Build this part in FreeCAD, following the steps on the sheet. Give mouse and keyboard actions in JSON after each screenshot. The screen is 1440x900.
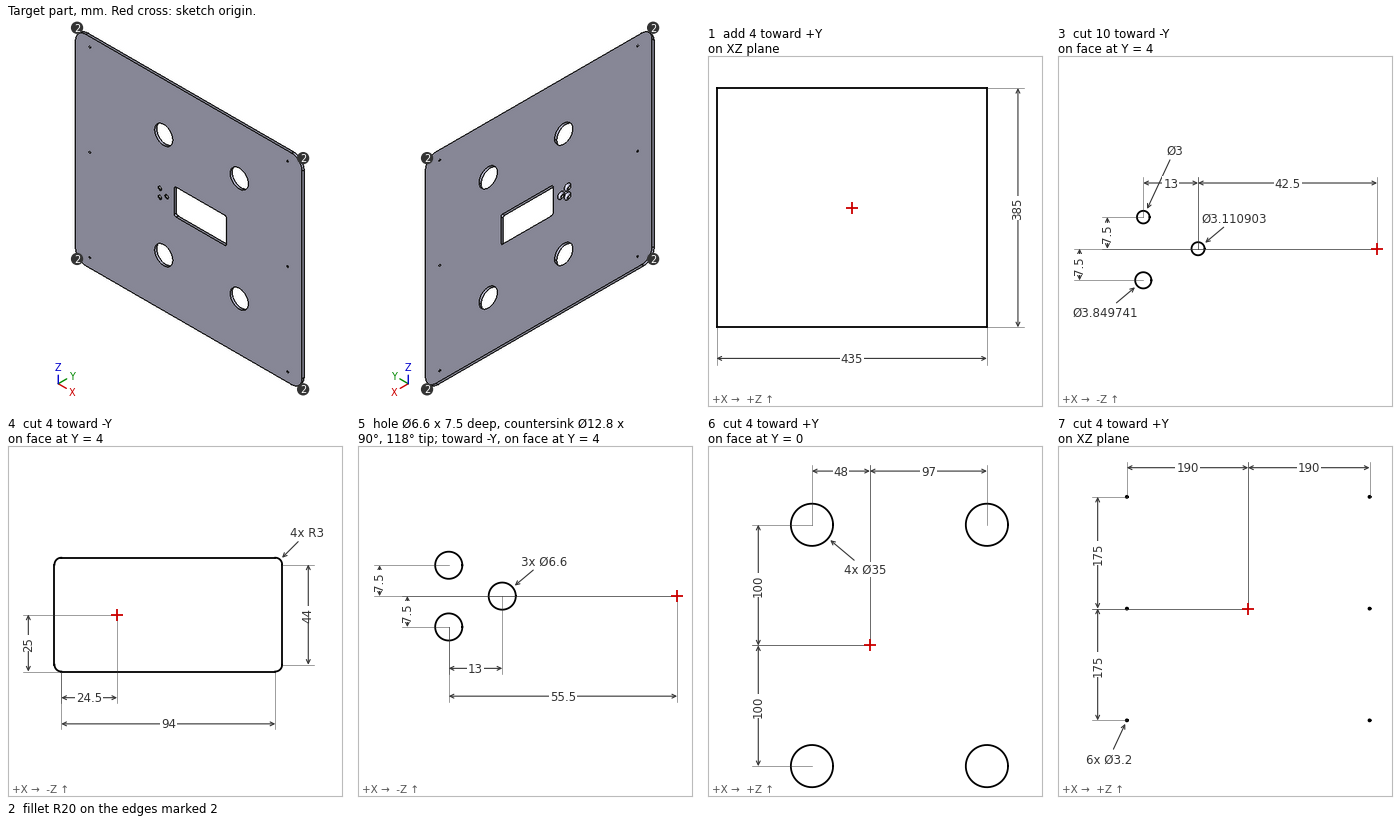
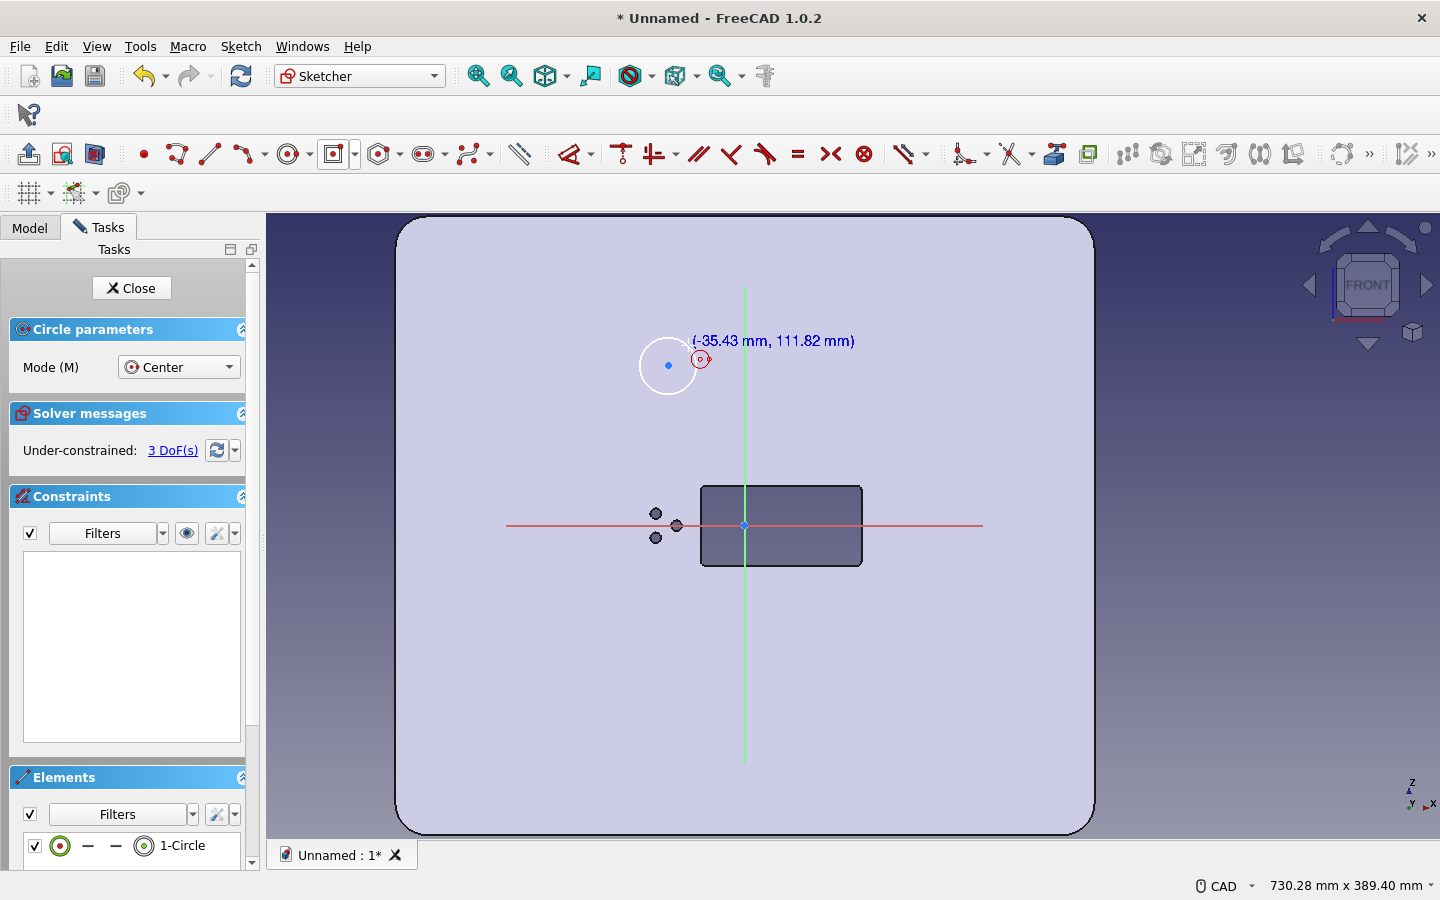
{"action": "left_click", "coordinate": [901, 365]}
{"action": "left_click", "coordinate": [921, 345]}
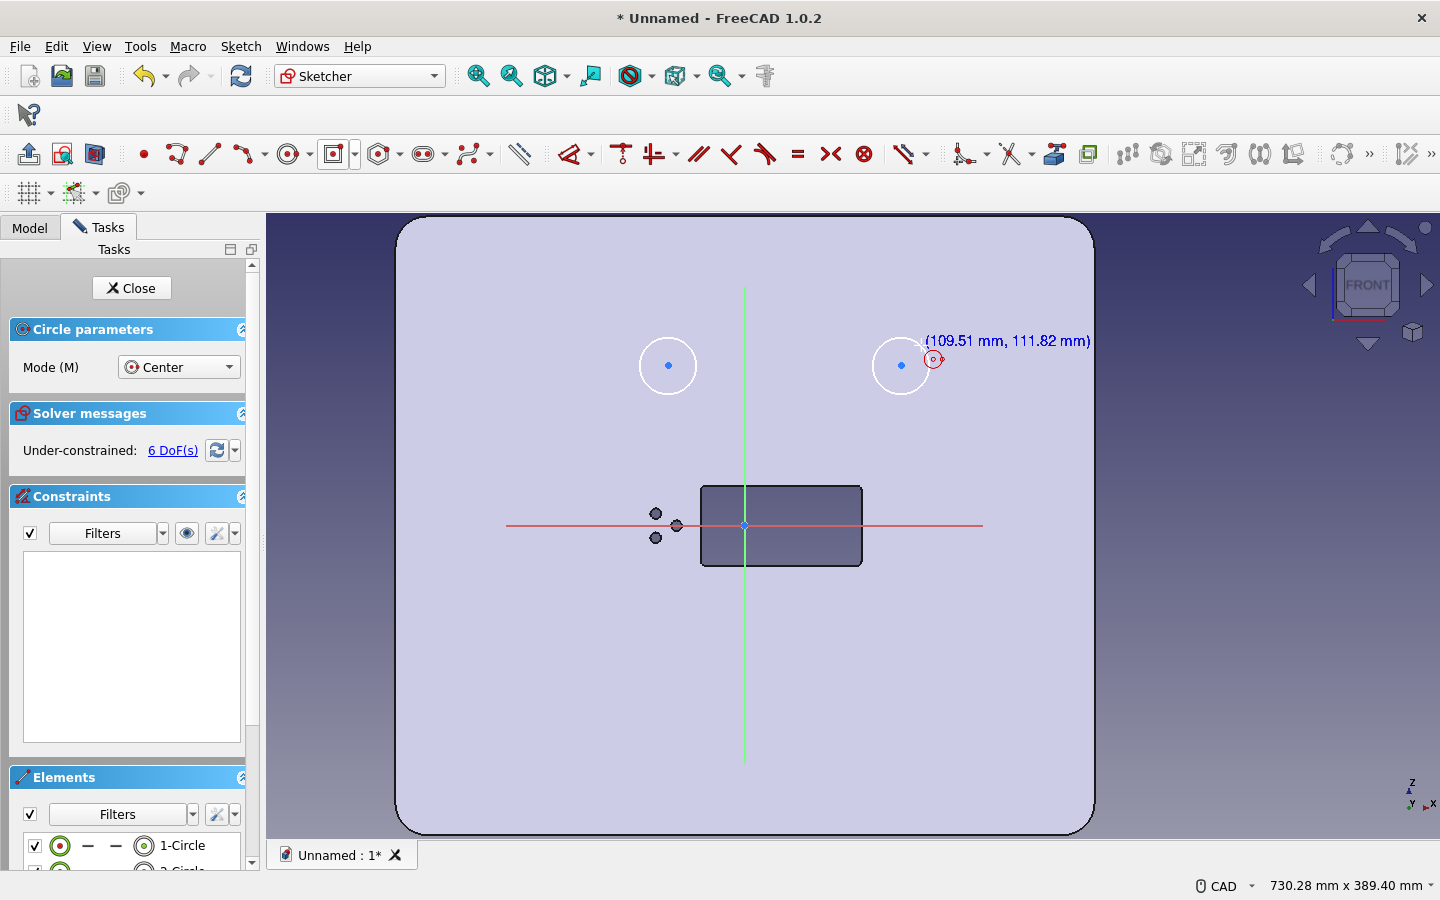
{"action": "left_click", "coordinate": [668, 687]}
{"action": "left_click", "coordinate": [688, 667]}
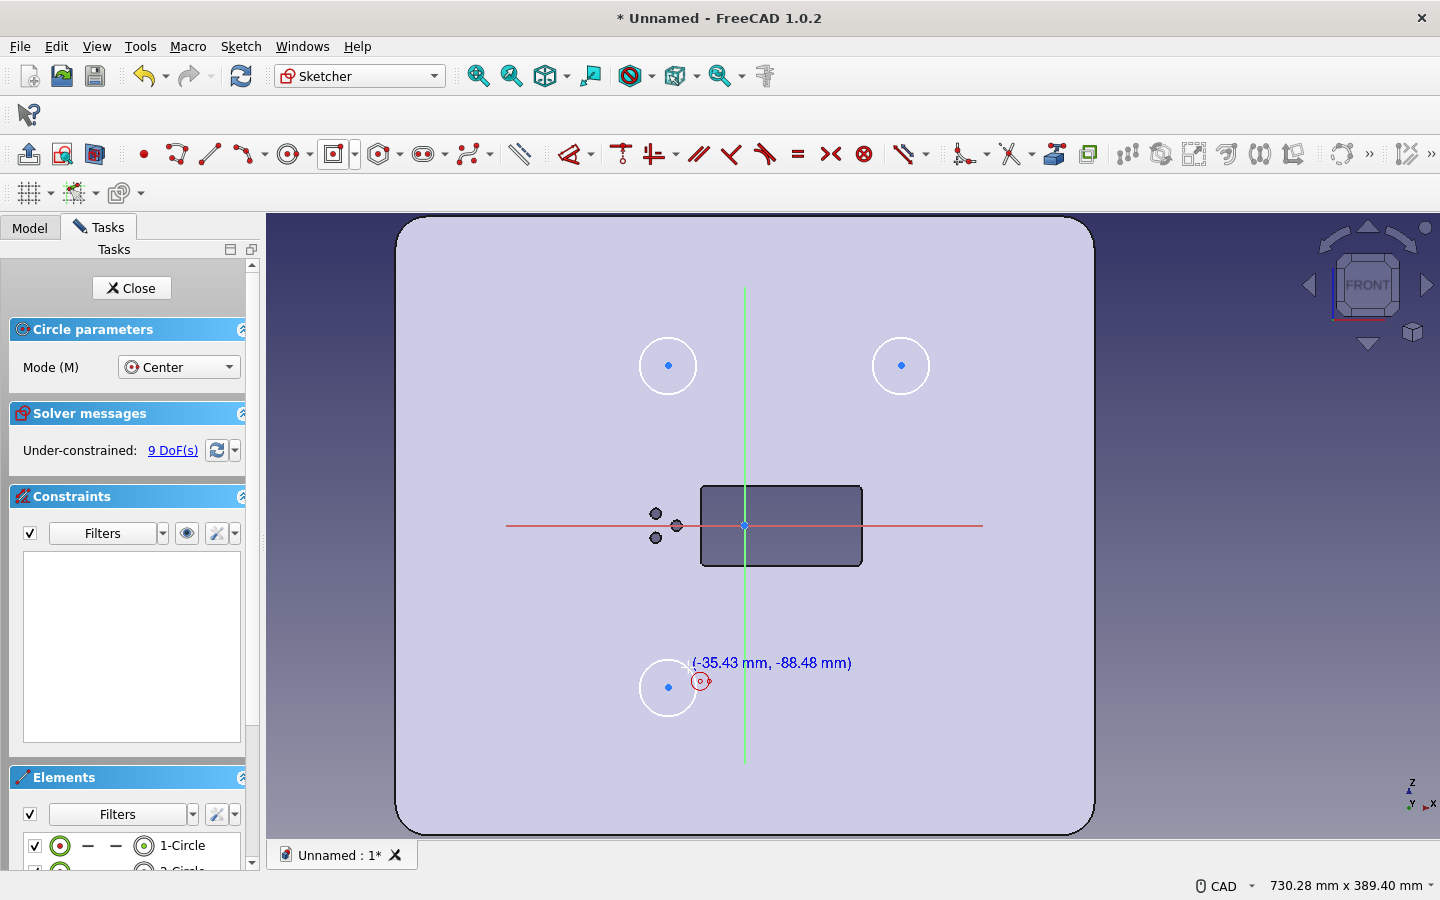
{"action": "left_click", "coordinate": [901, 687]}
{"action": "left_click", "coordinate": [921, 667]}
{"action": "key", "text": "Escape"}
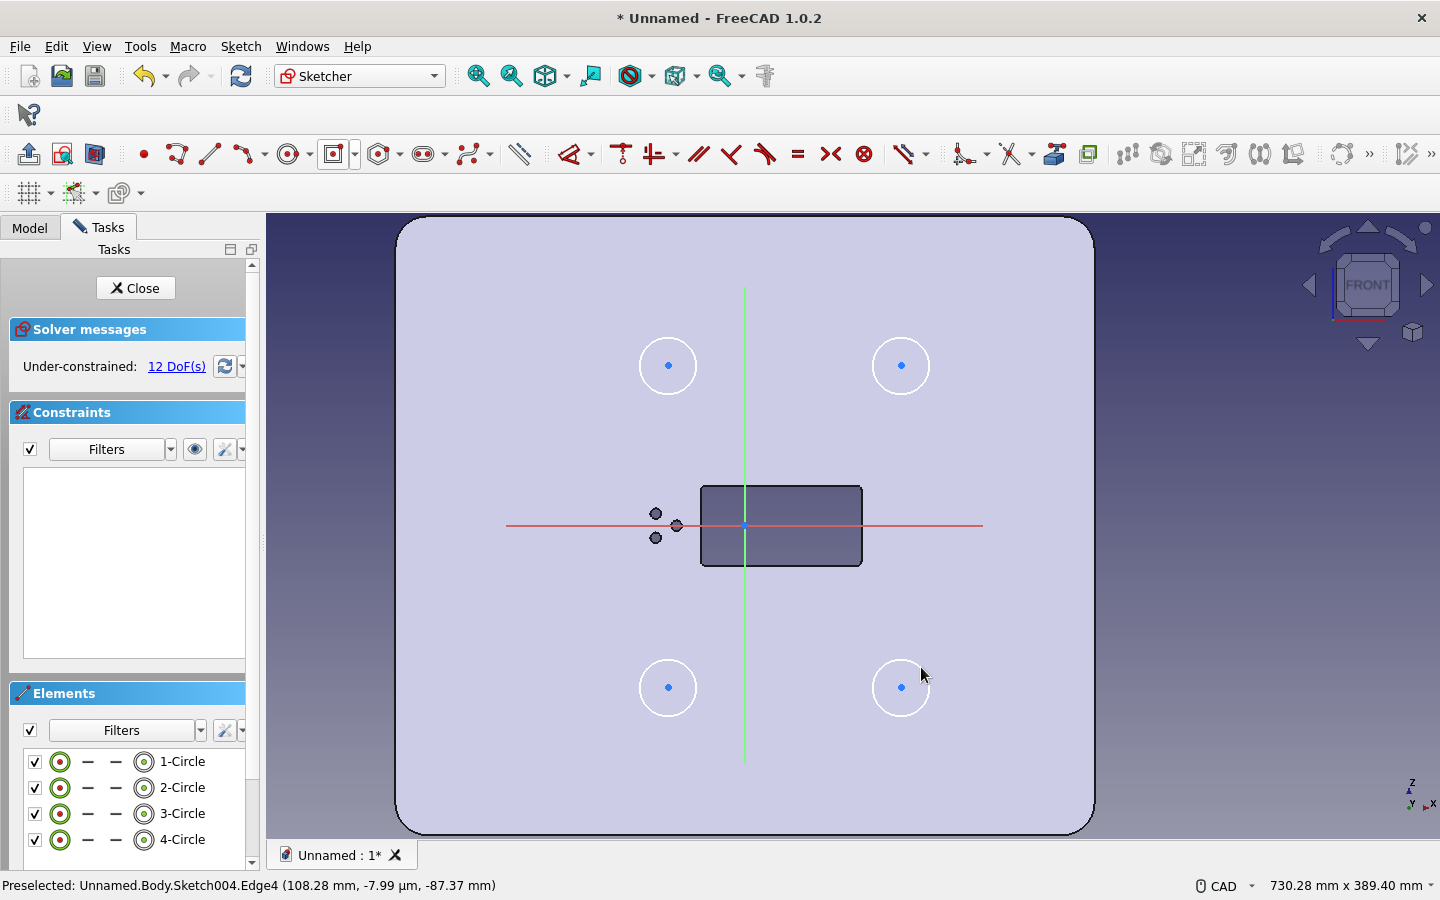
{"action": "left_click", "coordinate": [688, 346]}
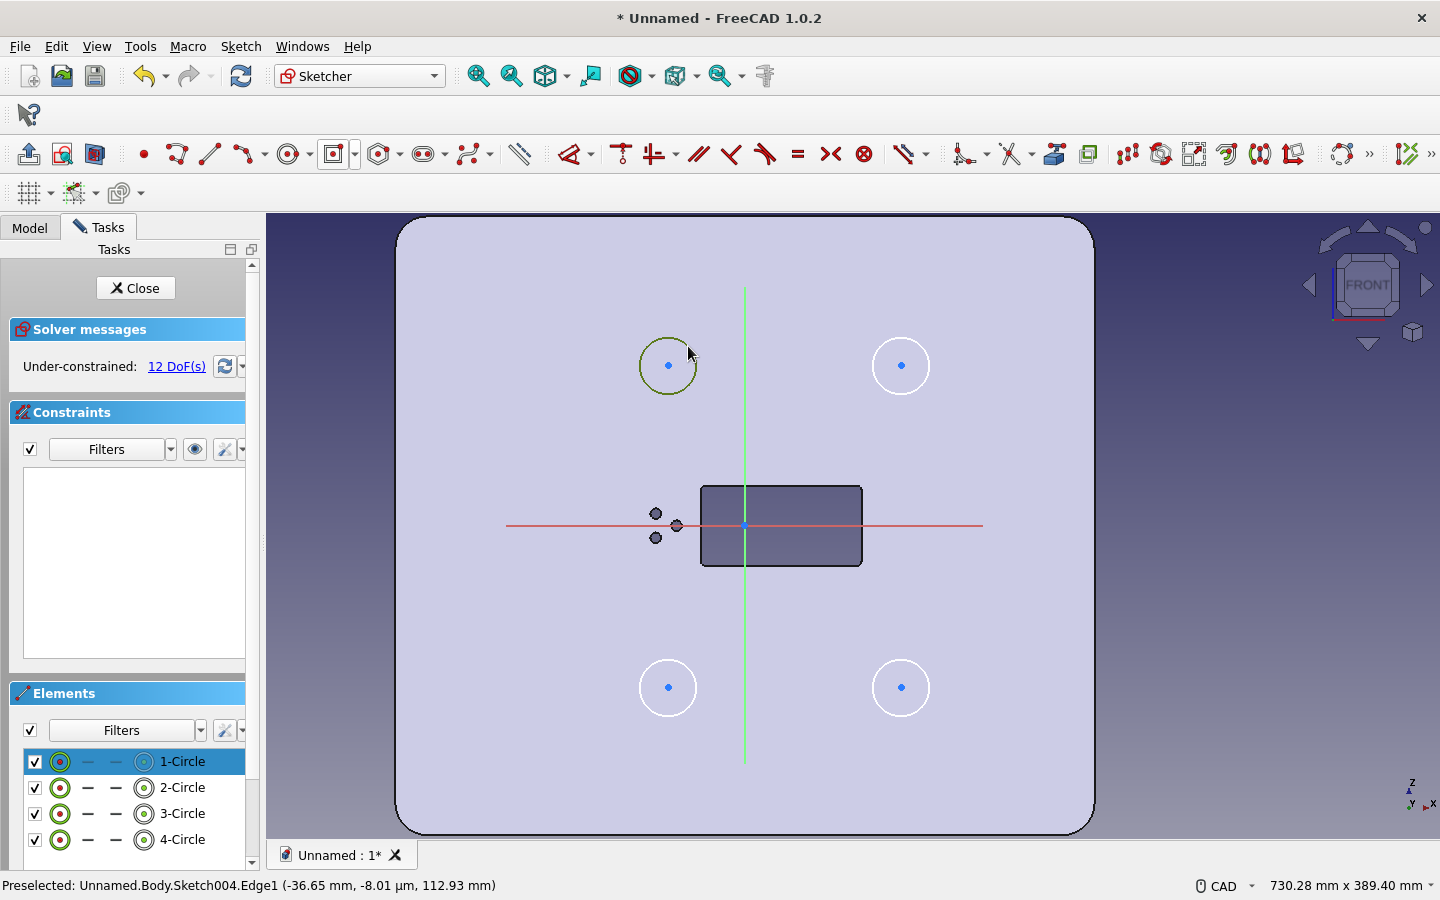
{"action": "left_click", "coordinate": [921, 346]}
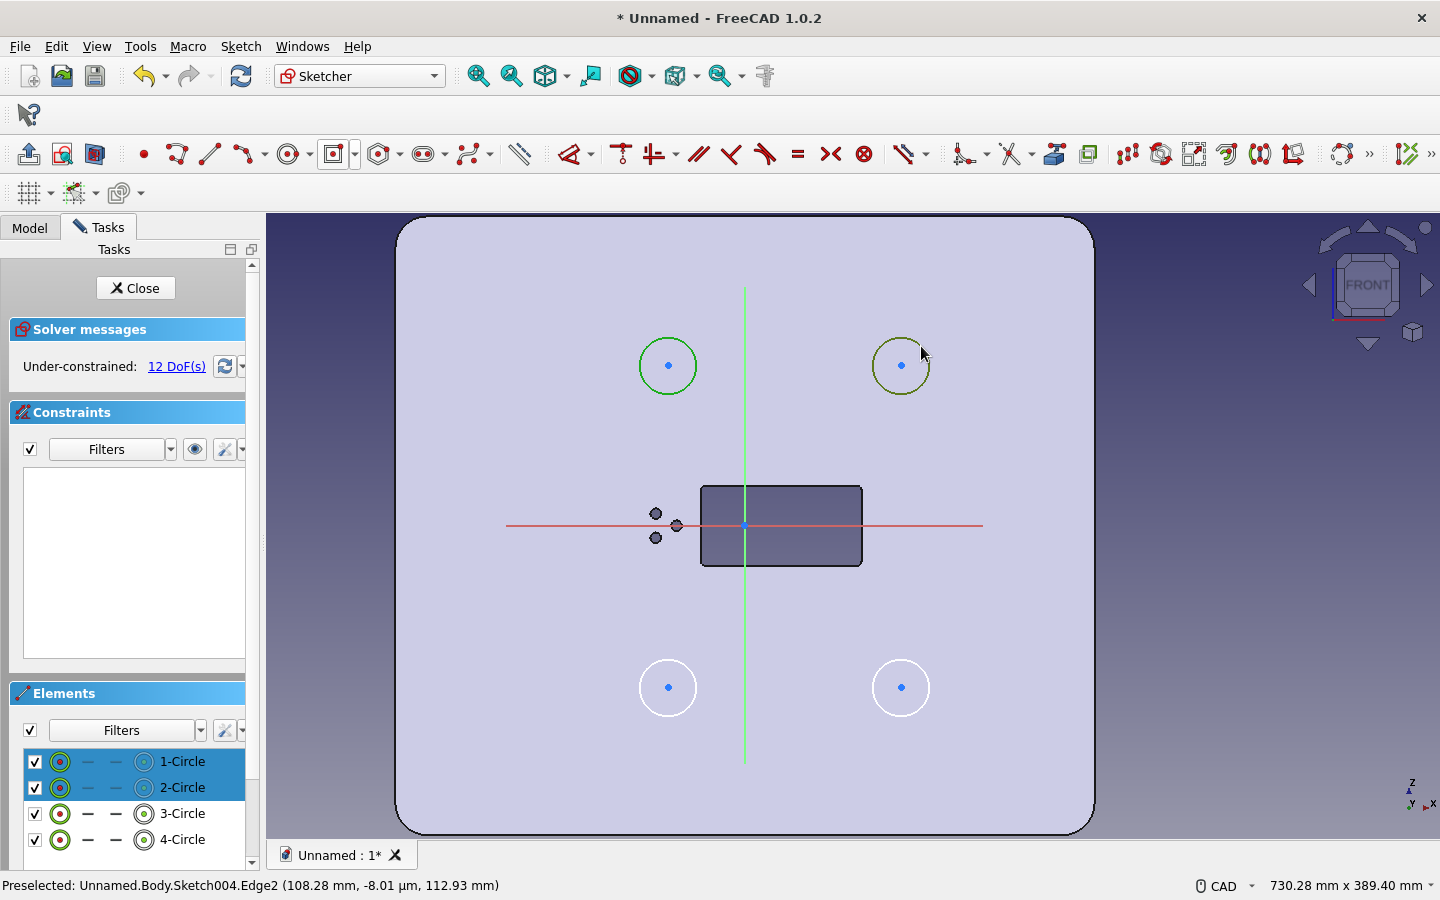
{"action": "left_click", "coordinate": [688, 668]}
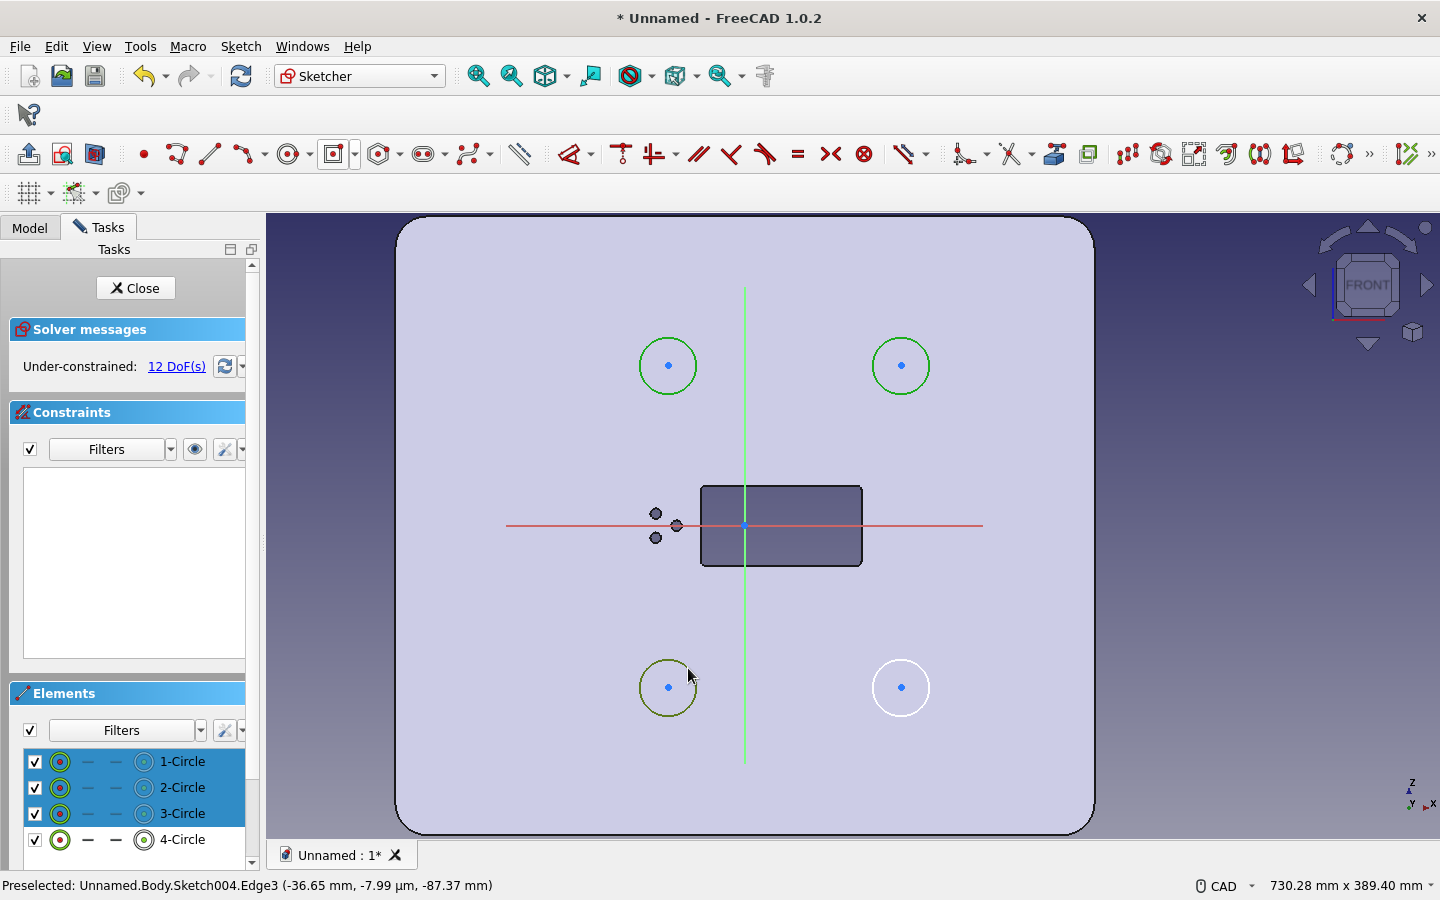
{"action": "left_click", "coordinate": [921, 668]}